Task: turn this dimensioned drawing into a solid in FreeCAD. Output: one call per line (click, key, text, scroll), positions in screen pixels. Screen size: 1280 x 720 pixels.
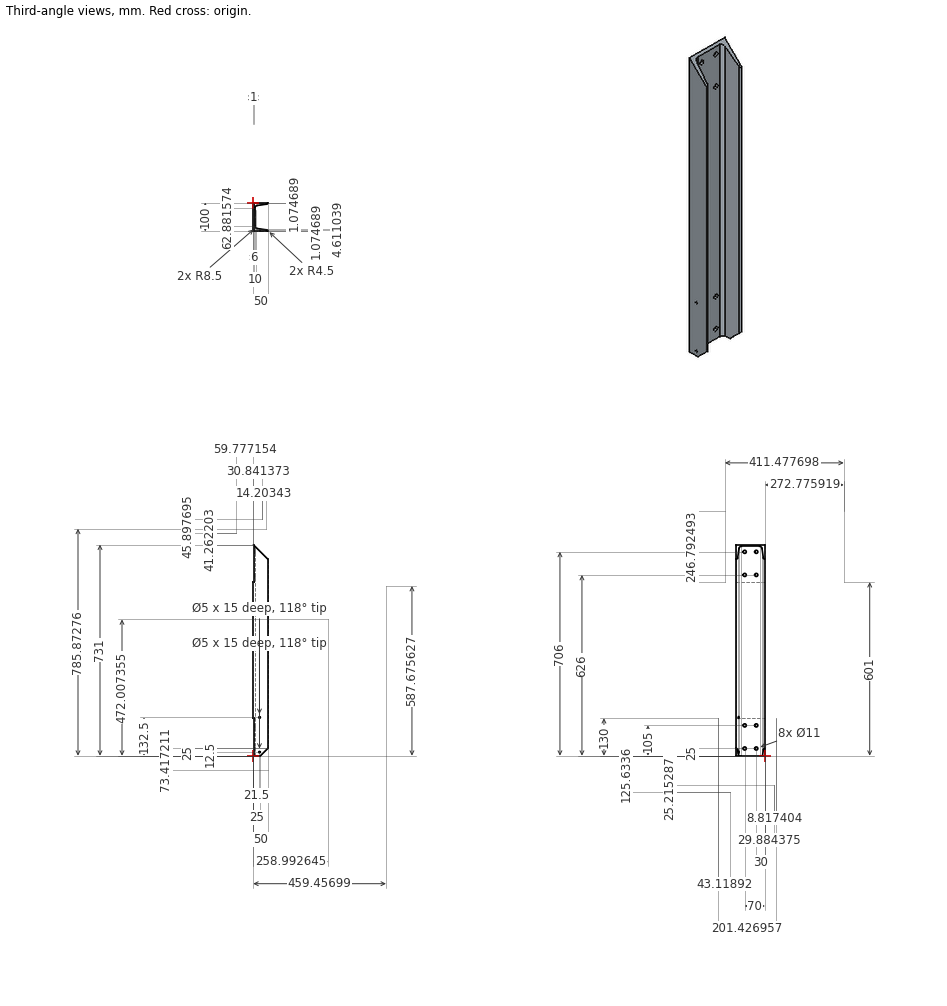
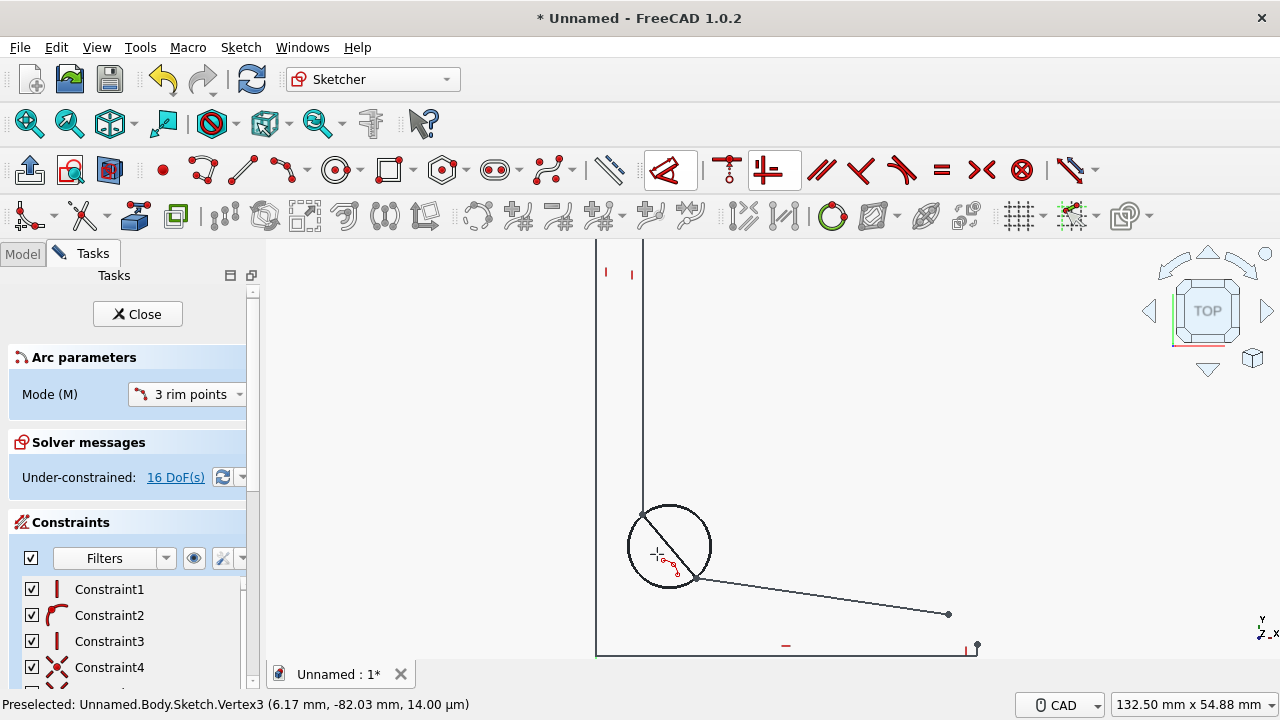
click(658, 553)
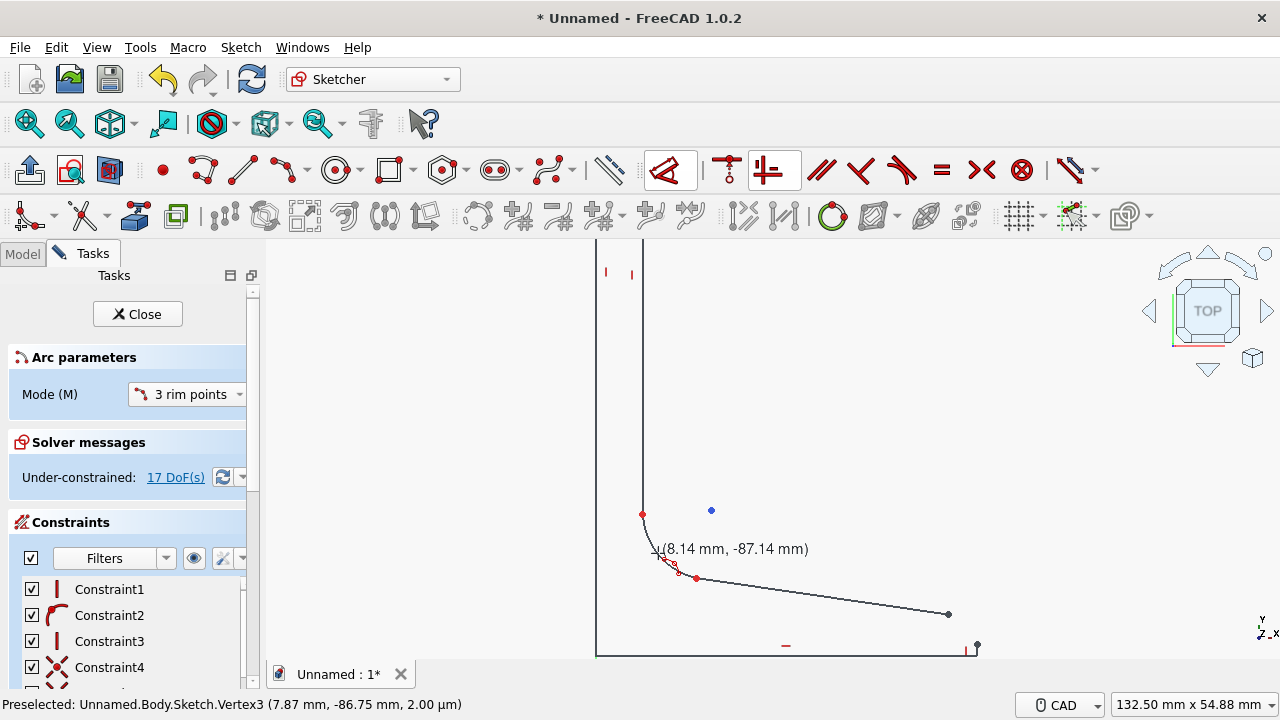
scroll(656, 553, down, 5)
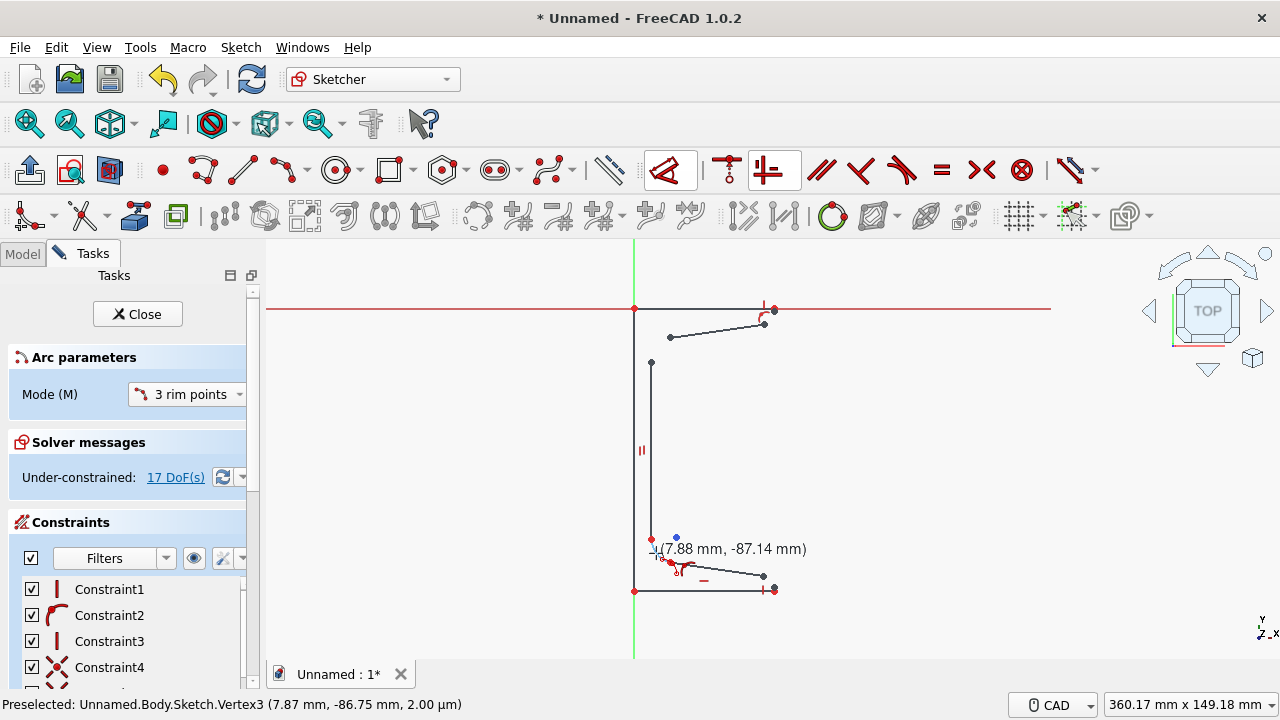
click(651, 362)
click(671, 338)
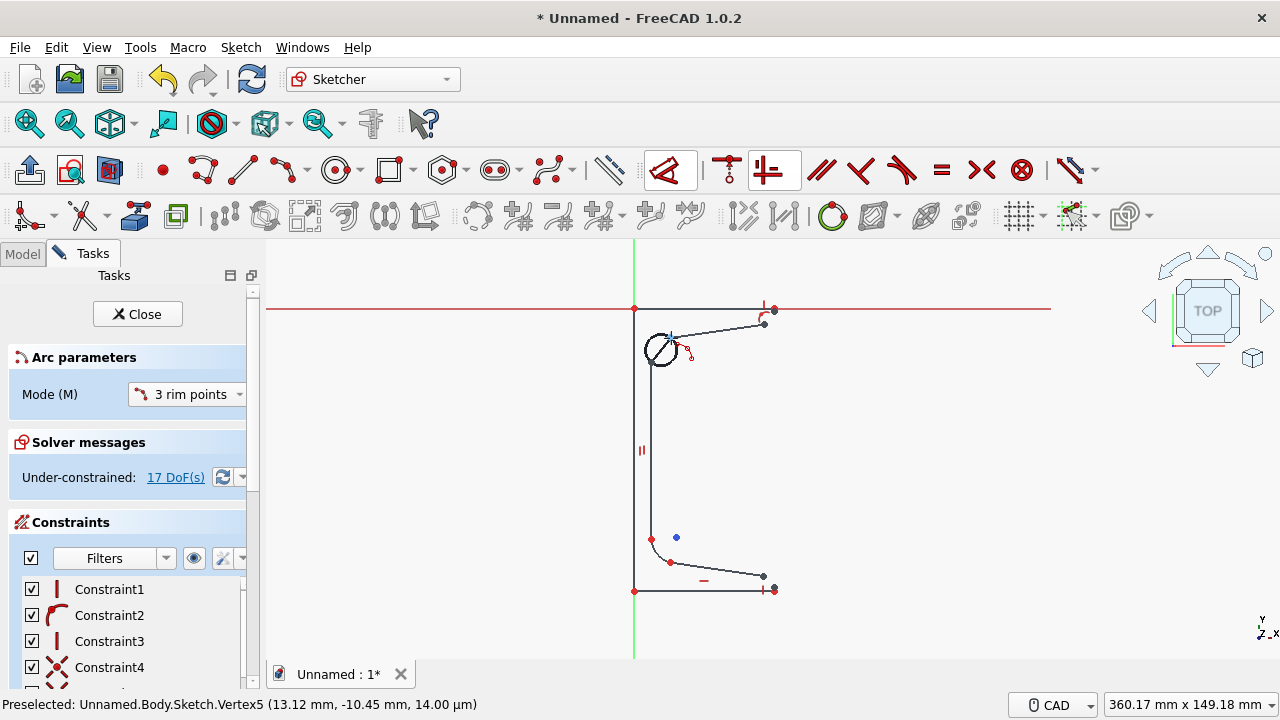
scroll(657, 345, up, 5)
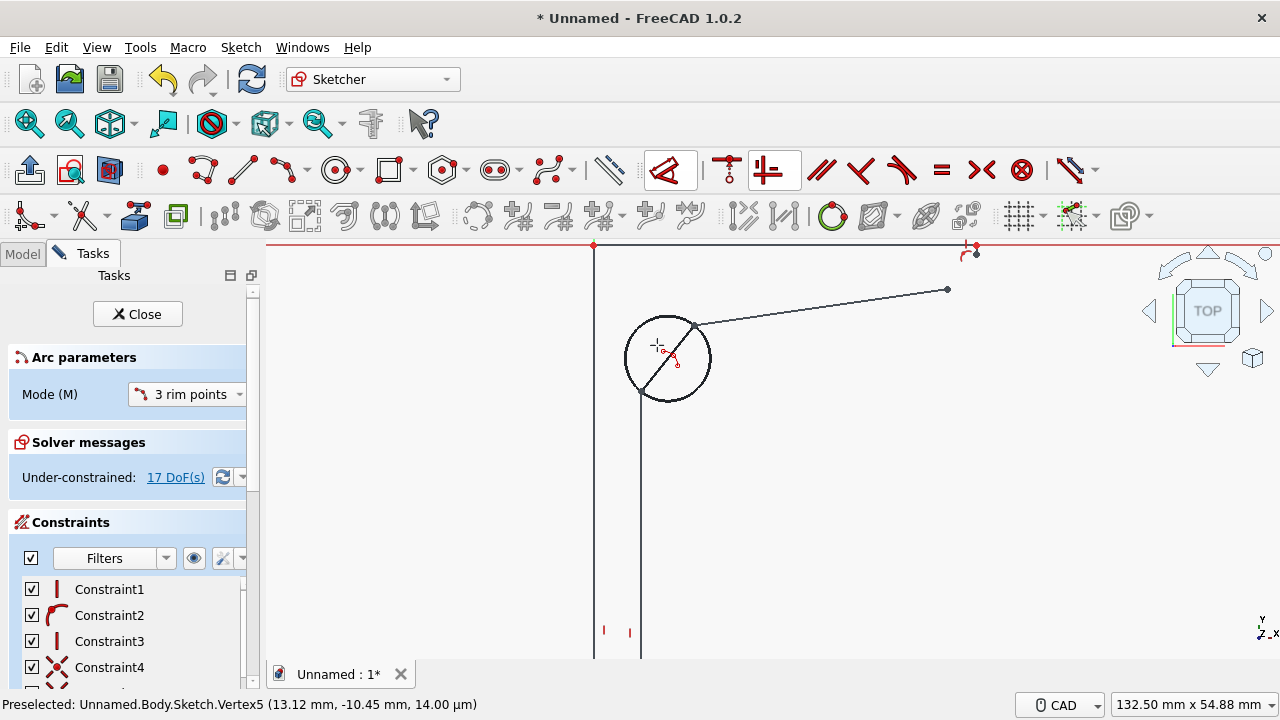
click(656, 345)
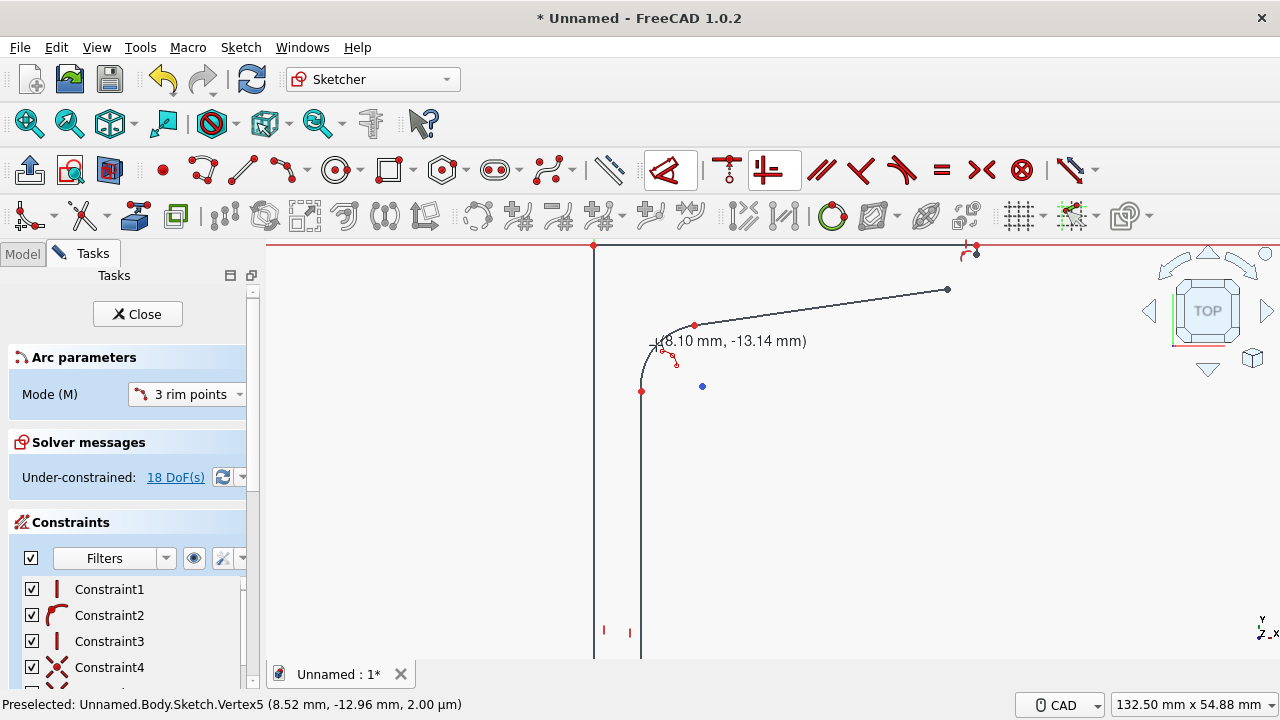
click(947, 289)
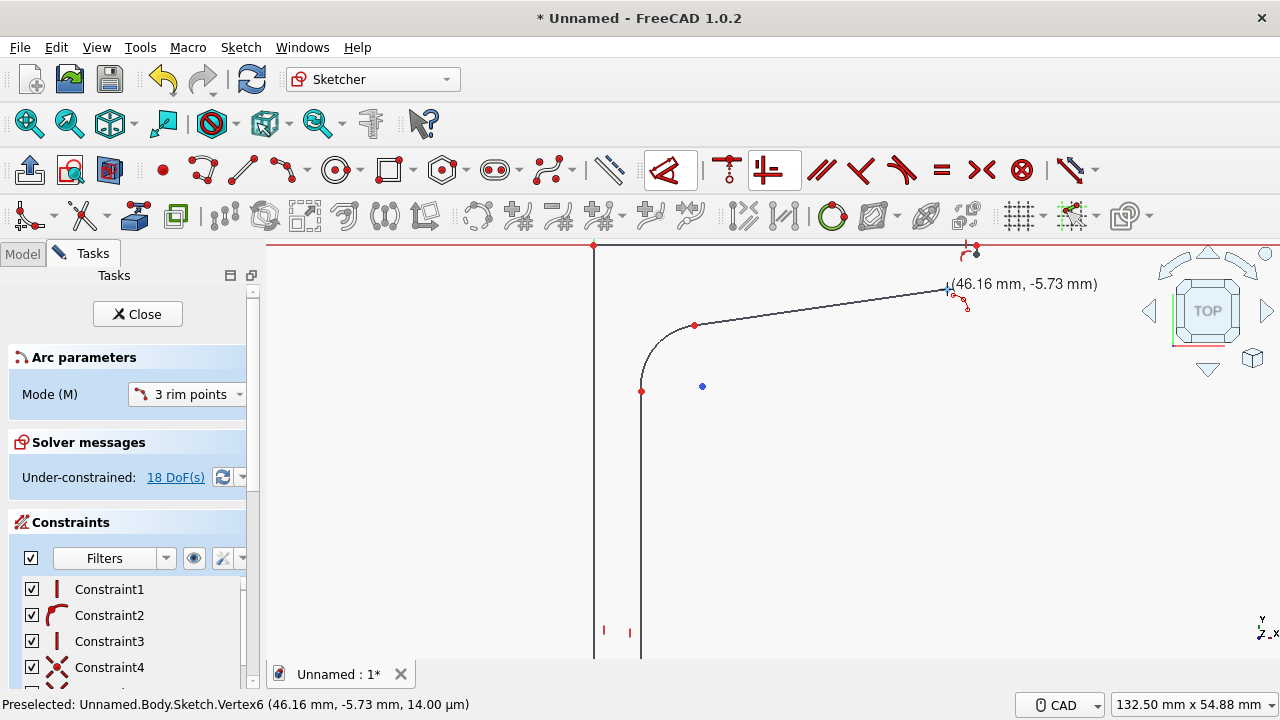
scroll(657, 345, down, 5)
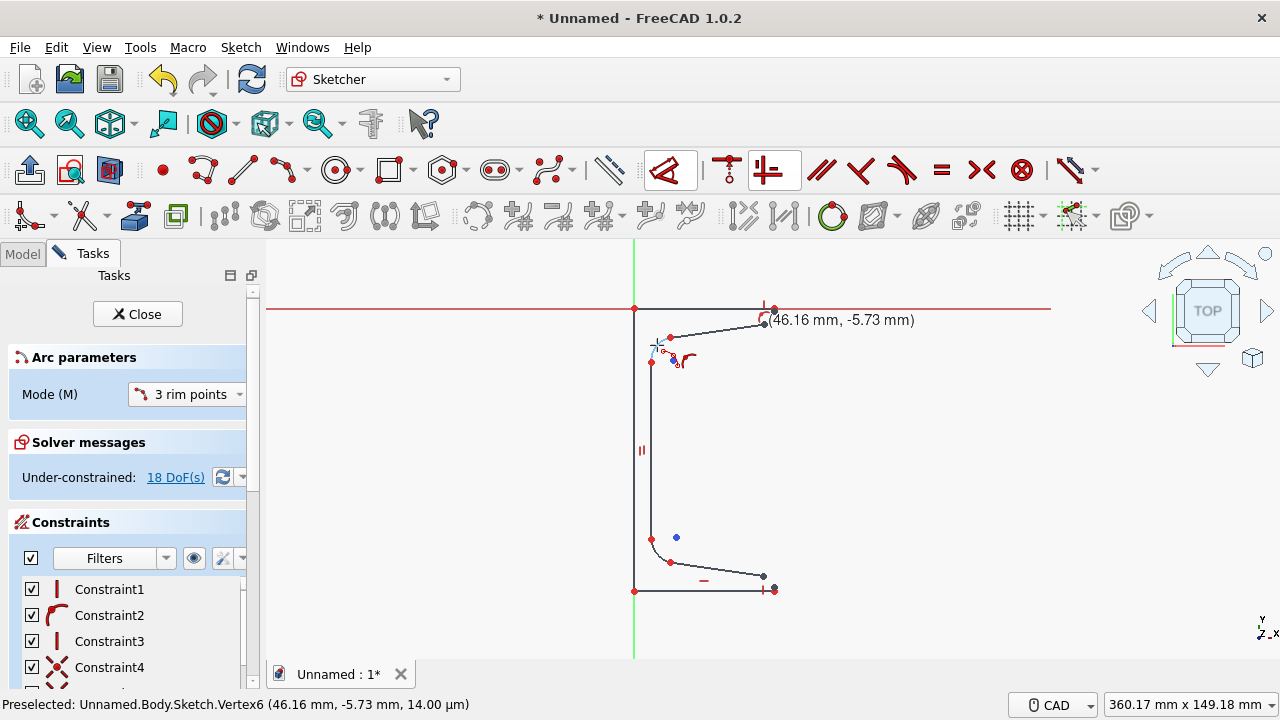
scroll(775, 312, up, 12)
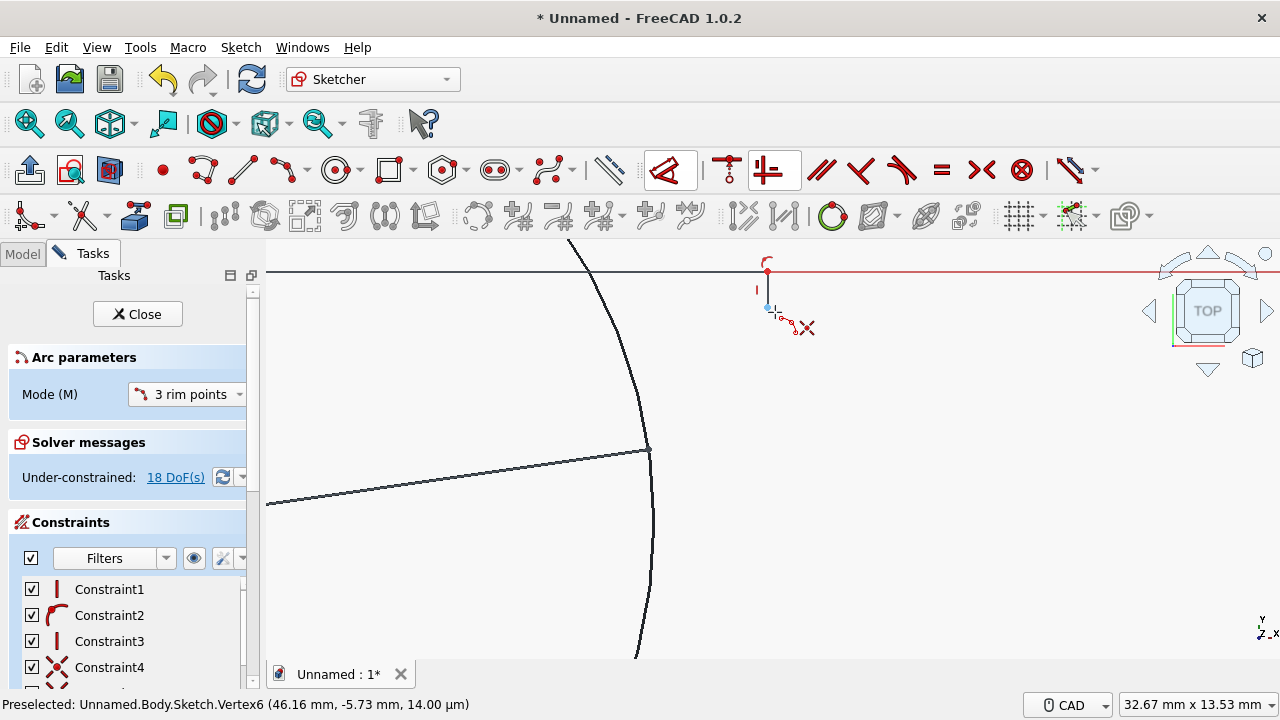
click(768, 307)
click(734, 397)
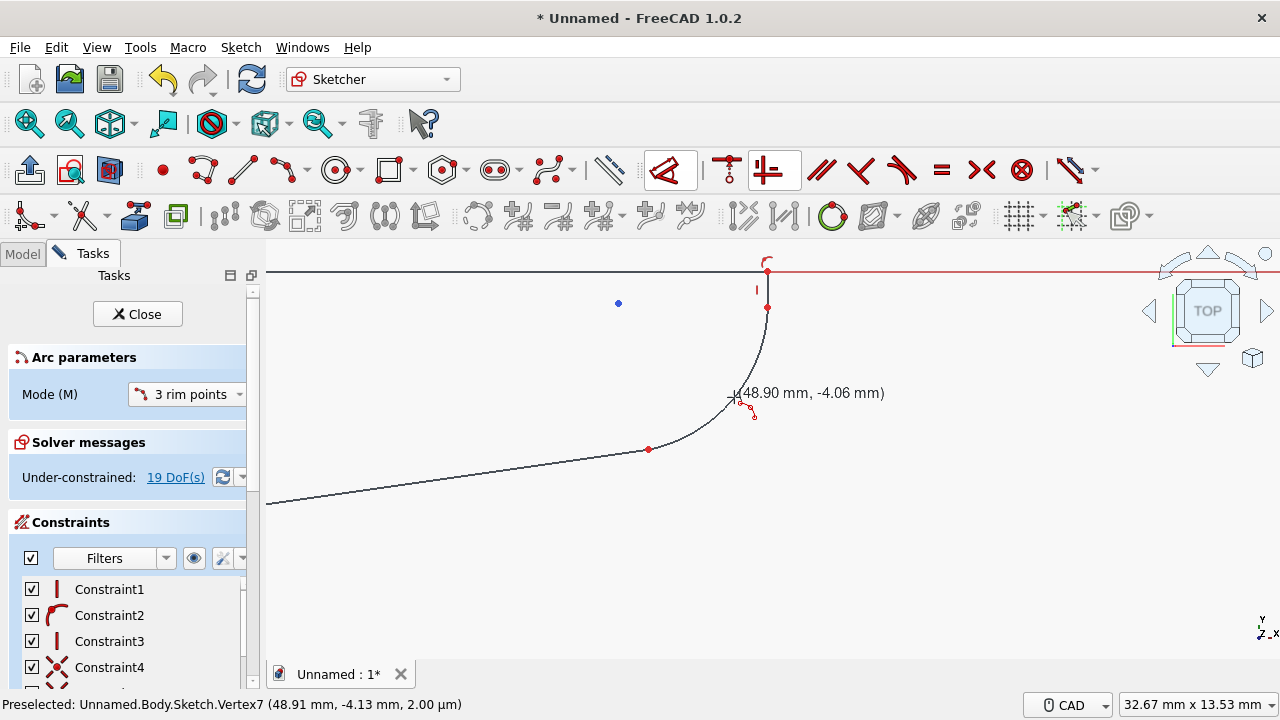
scroll(776, 312, down, 12)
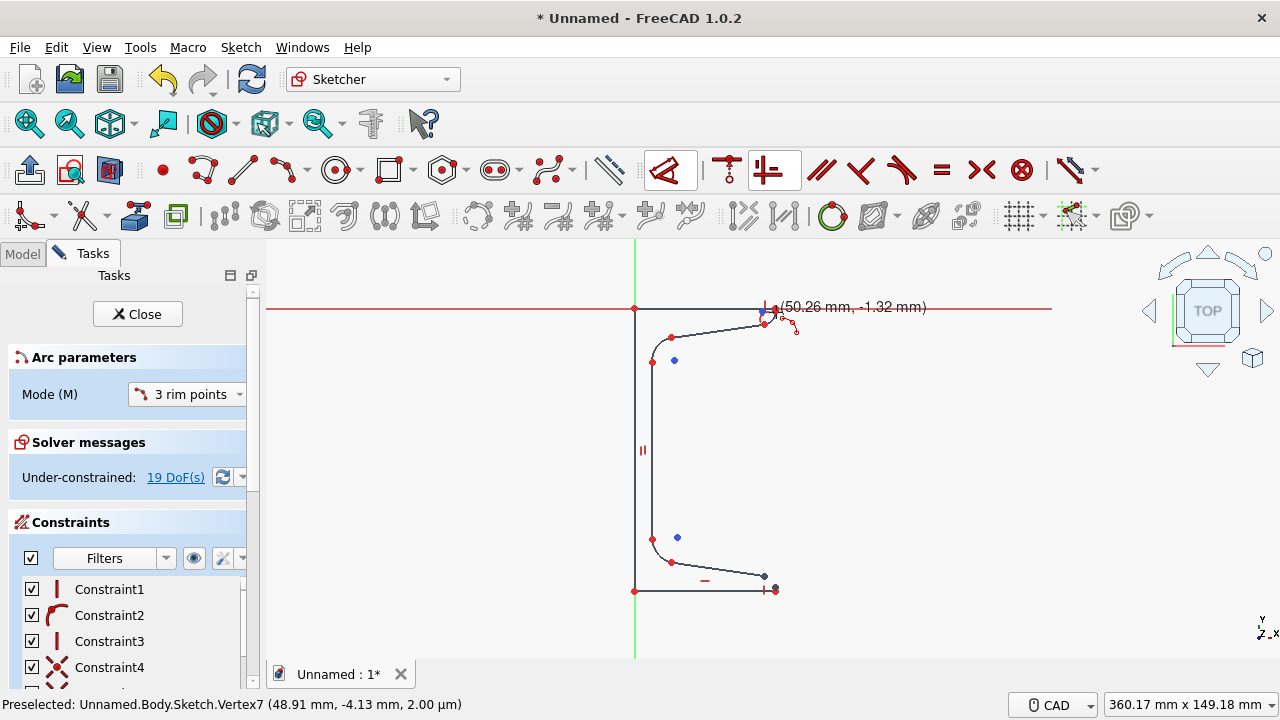
scroll(776, 587, up, 12)